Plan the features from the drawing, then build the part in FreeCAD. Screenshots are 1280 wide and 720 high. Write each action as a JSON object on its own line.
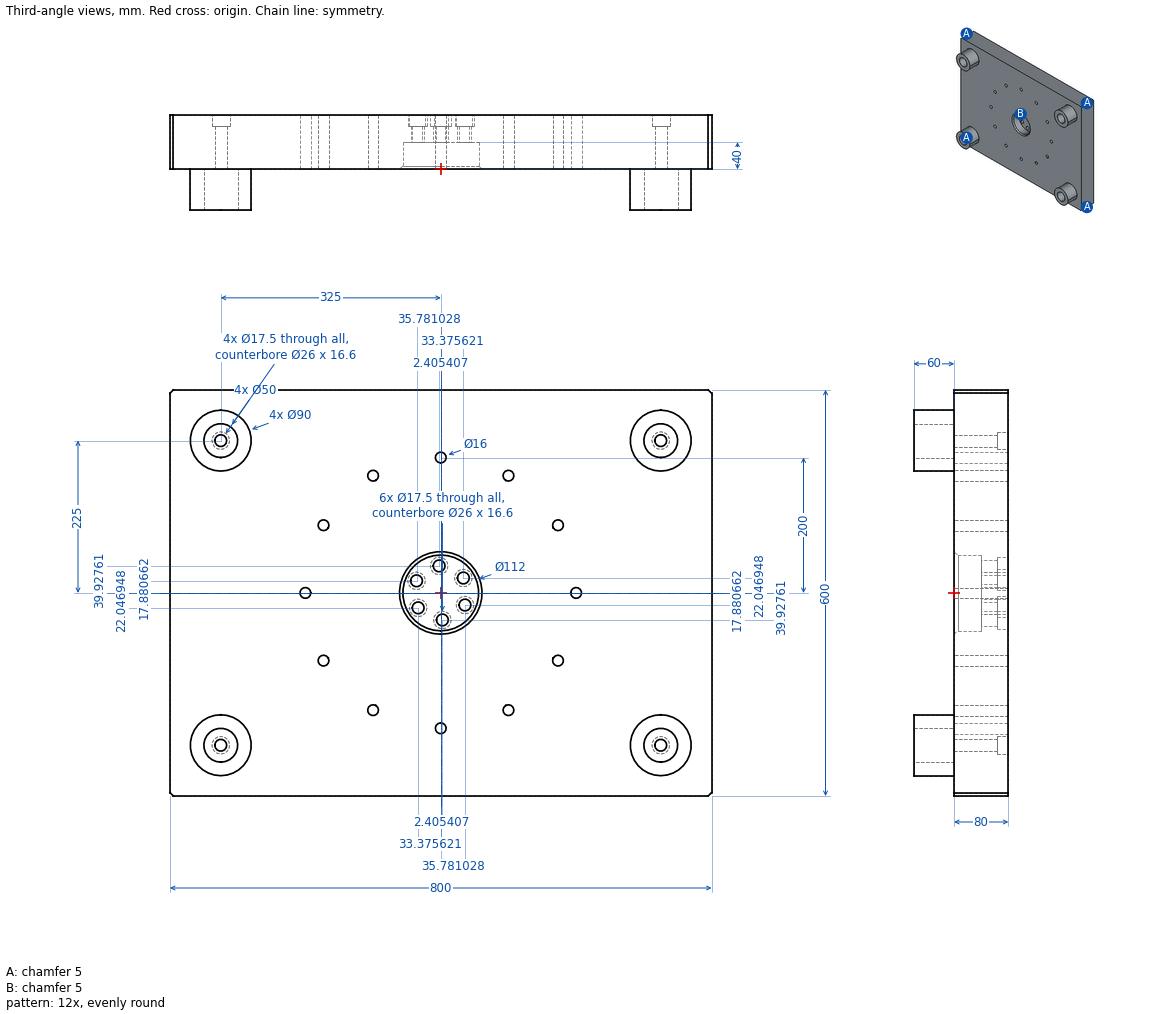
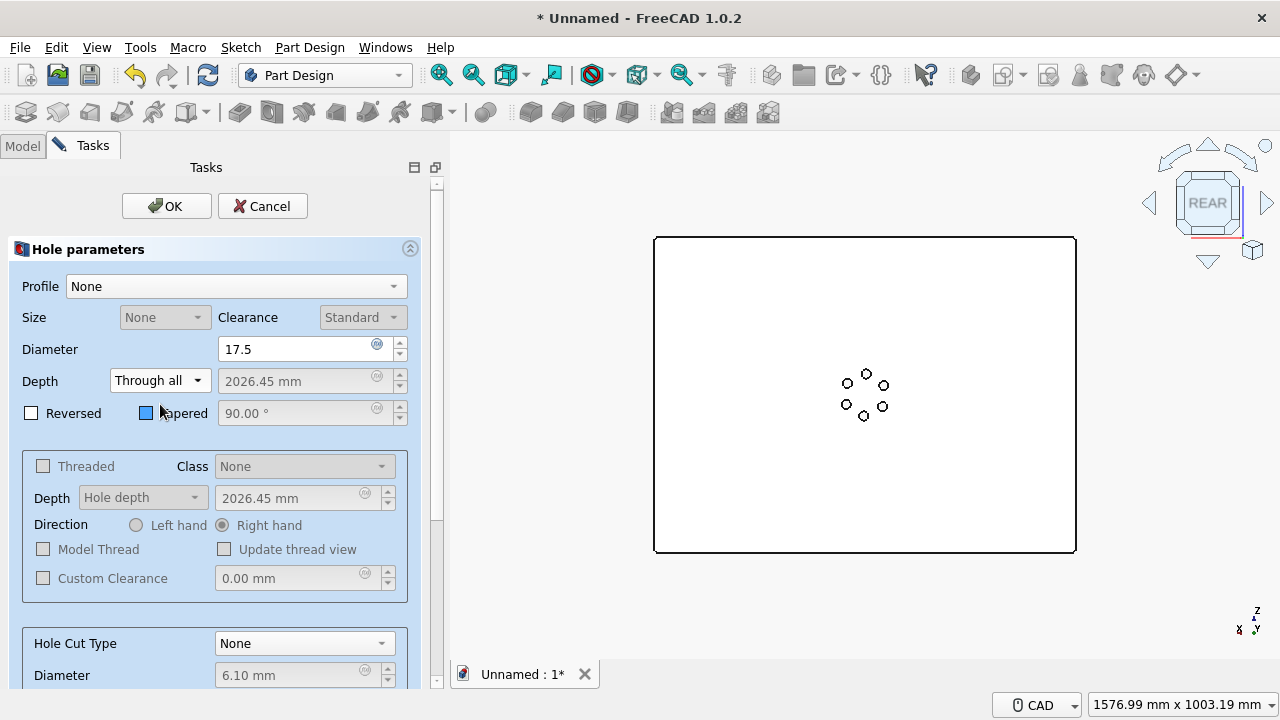
{"action": "left_click", "coordinate": [306, 644]}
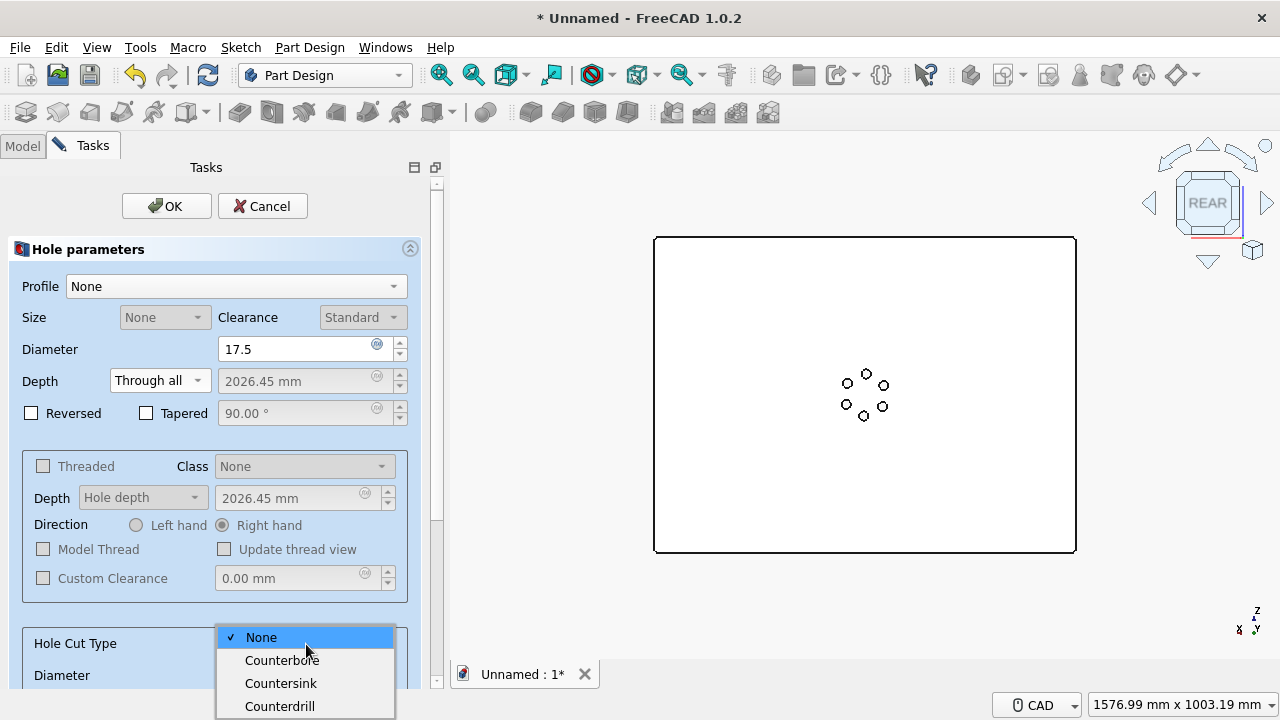
{"action": "left_click", "coordinate": [304, 660]}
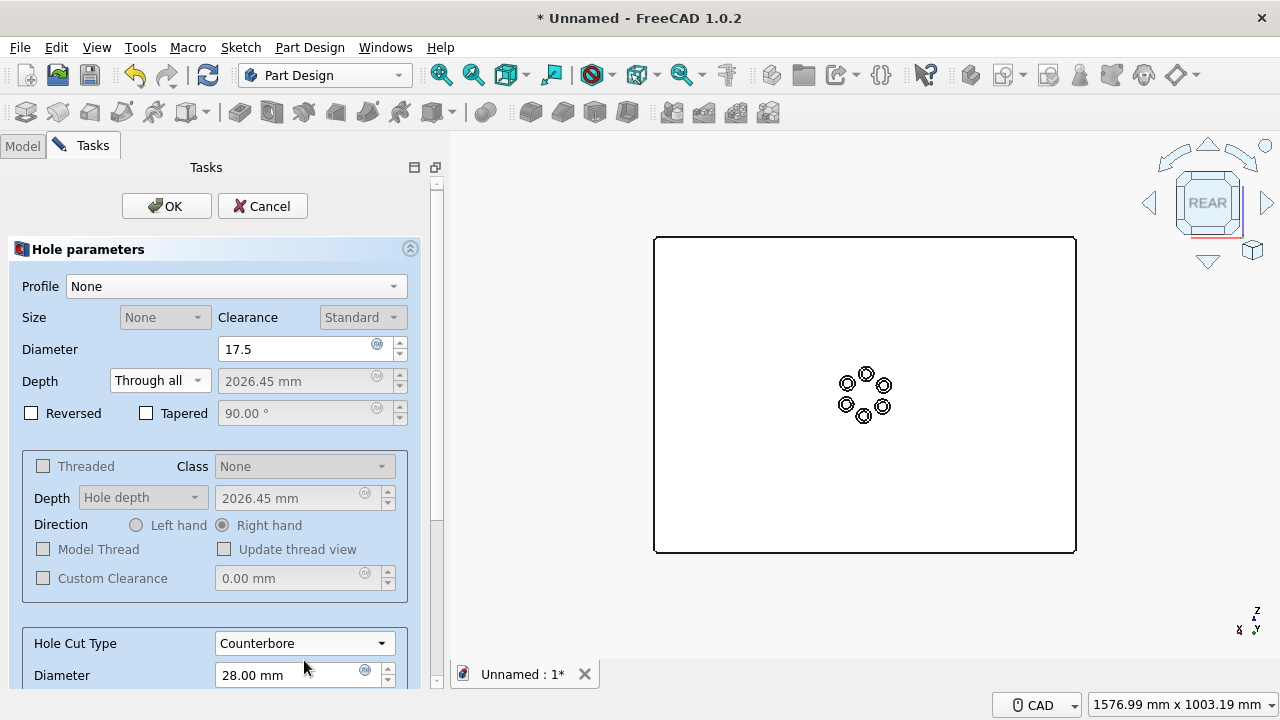
{"action": "triple_click", "coordinate": [298, 675]}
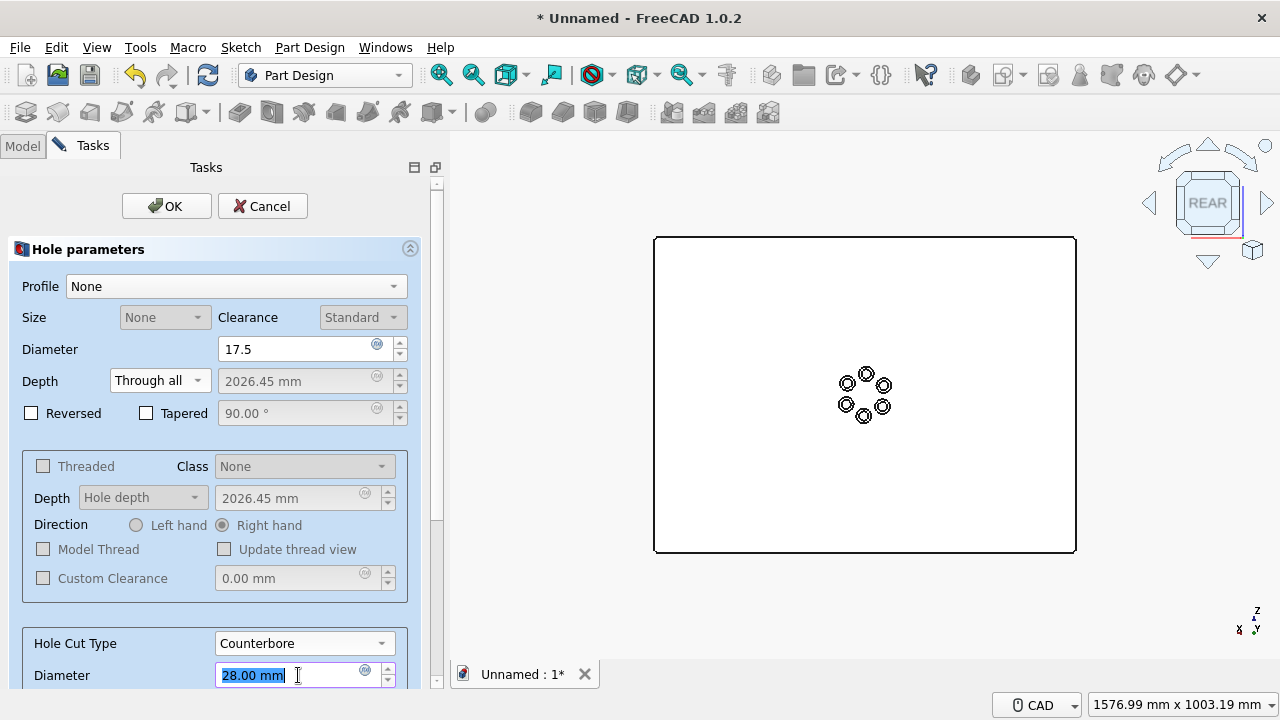
{"action": "type", "text": "26"}
{"action": "key", "text": "Tab"}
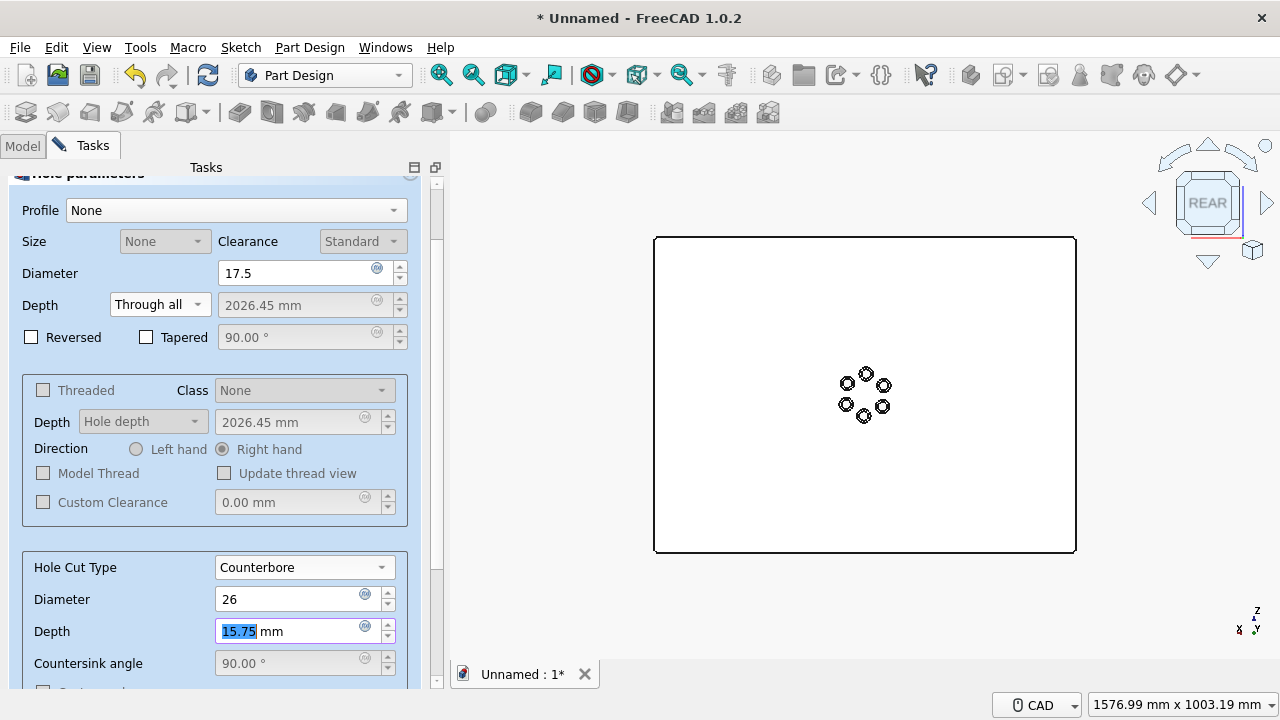
{"action": "type", "text": "16.6"}
{"action": "key", "text": "Tab"}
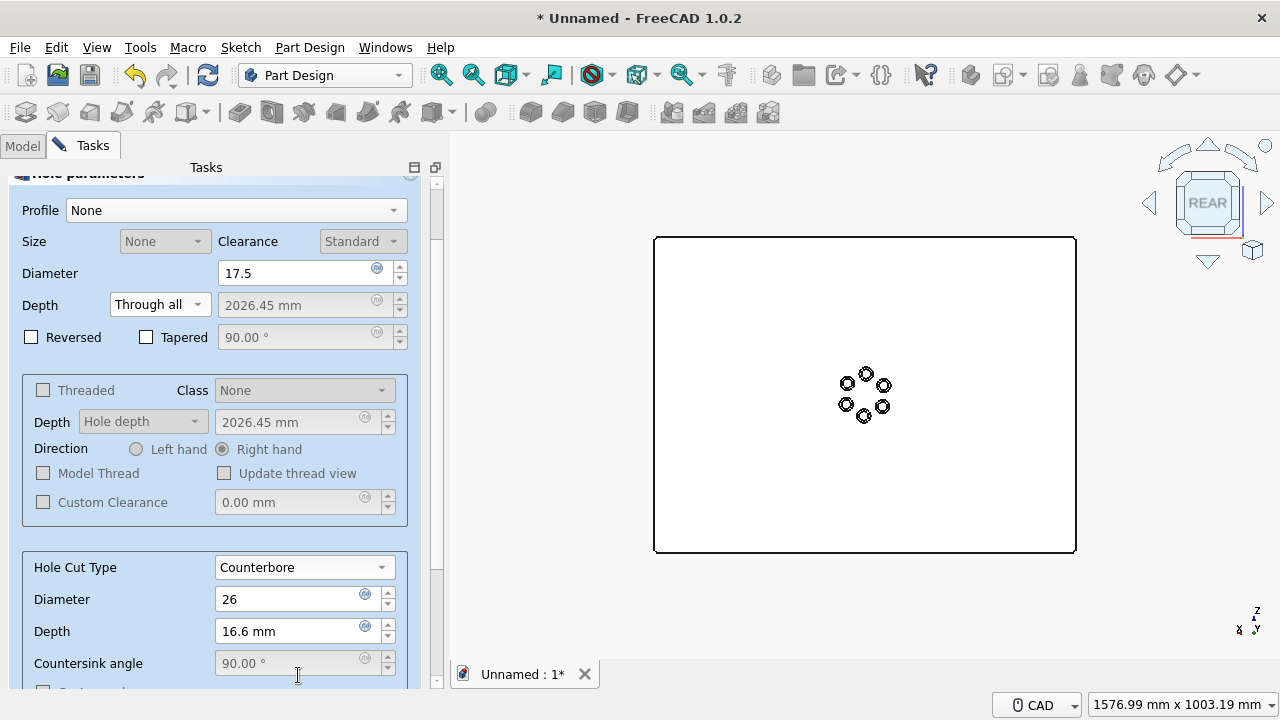
{"action": "scroll", "coordinate": [437, 432], "scroll_direction": "up", "scroll_amount": 3}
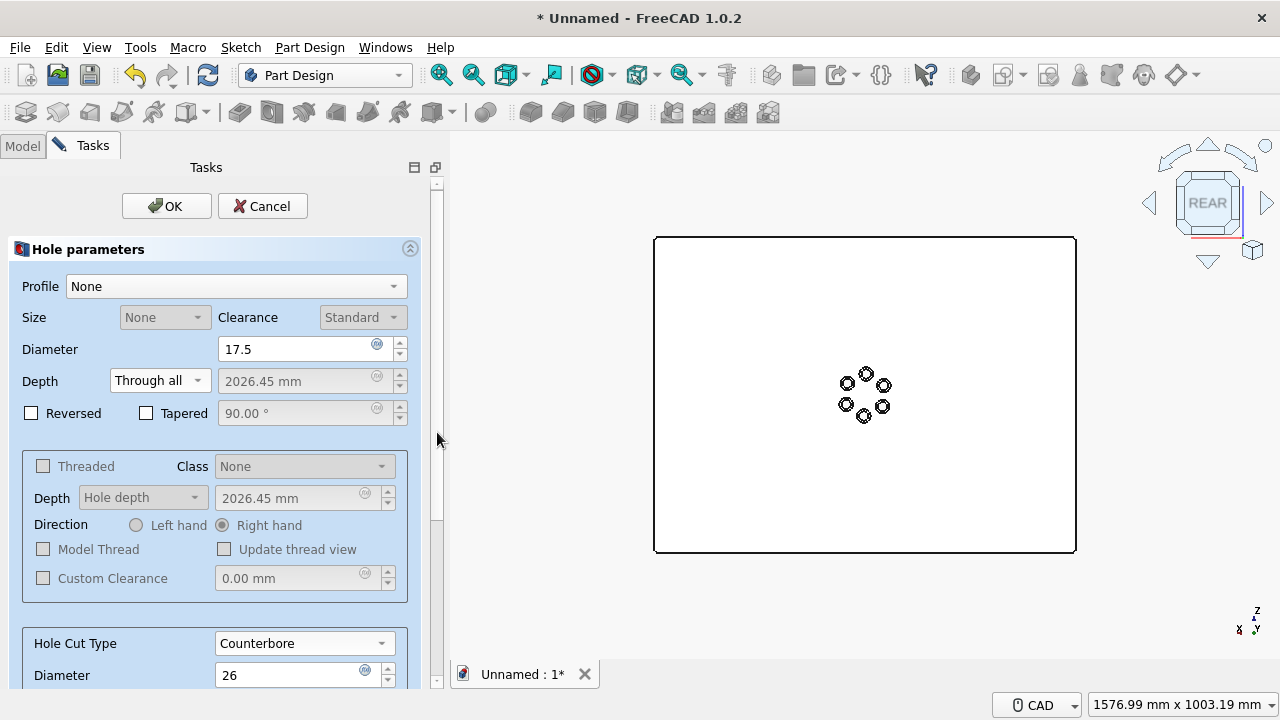
{"action": "left_click", "coordinate": [167, 206]}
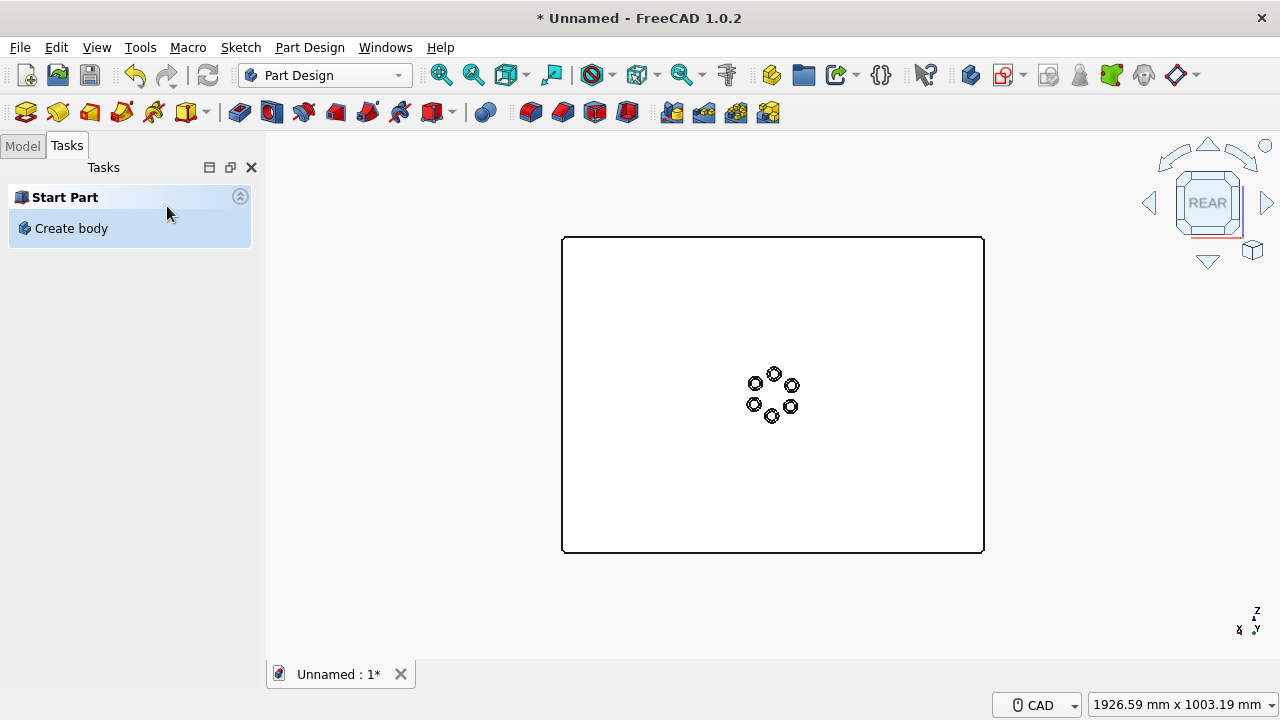
{"action": "key", "text": "0"}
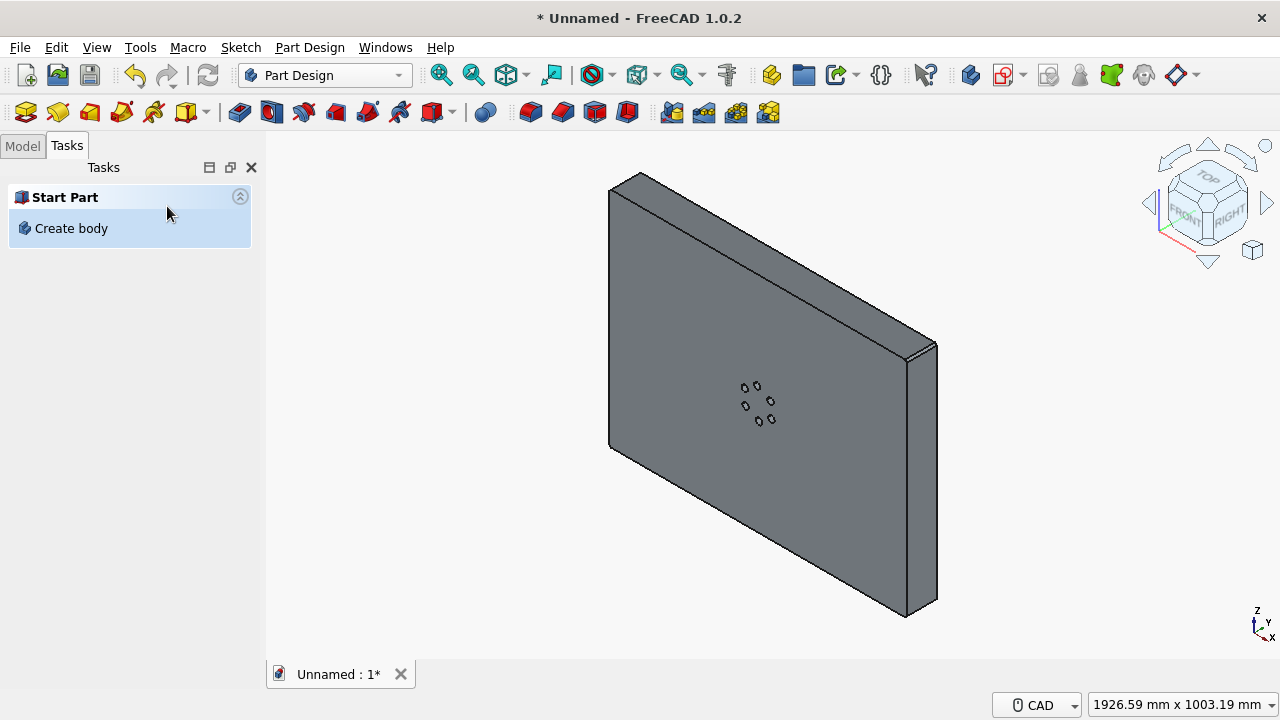
{"action": "left_click", "coordinate": [843, 415]}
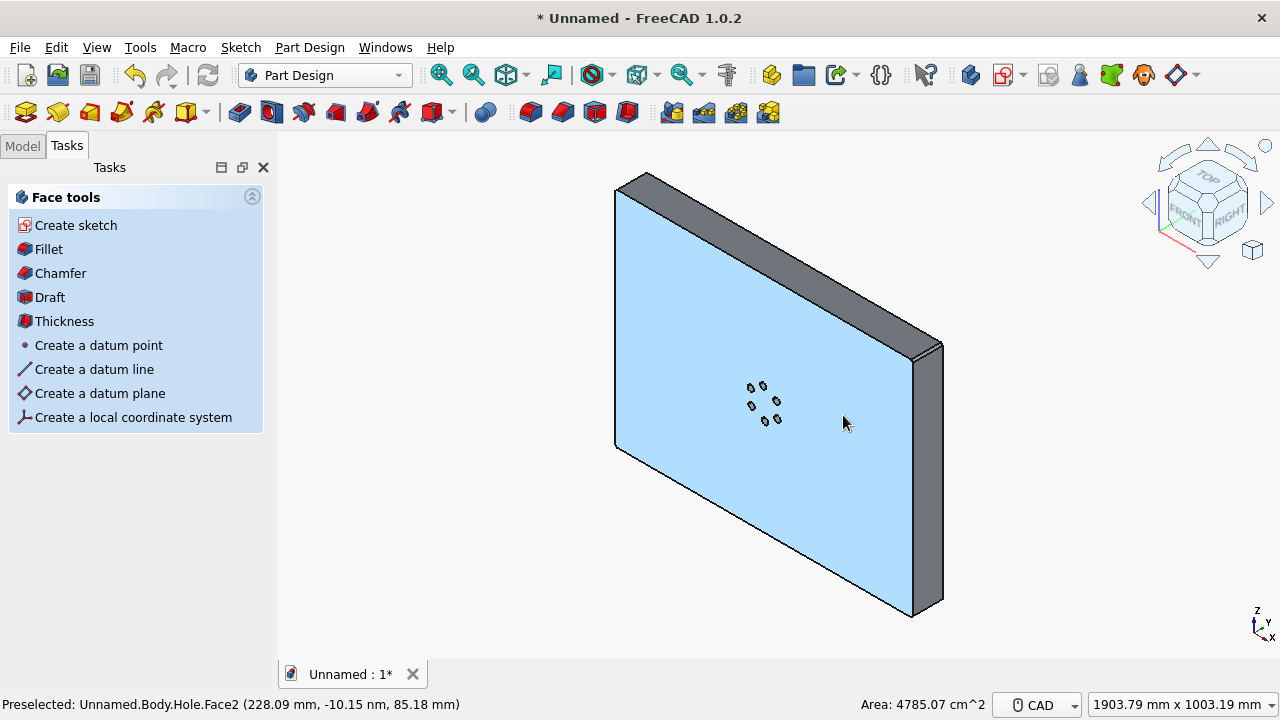
{"action": "left_click", "coordinate": [1004, 76]}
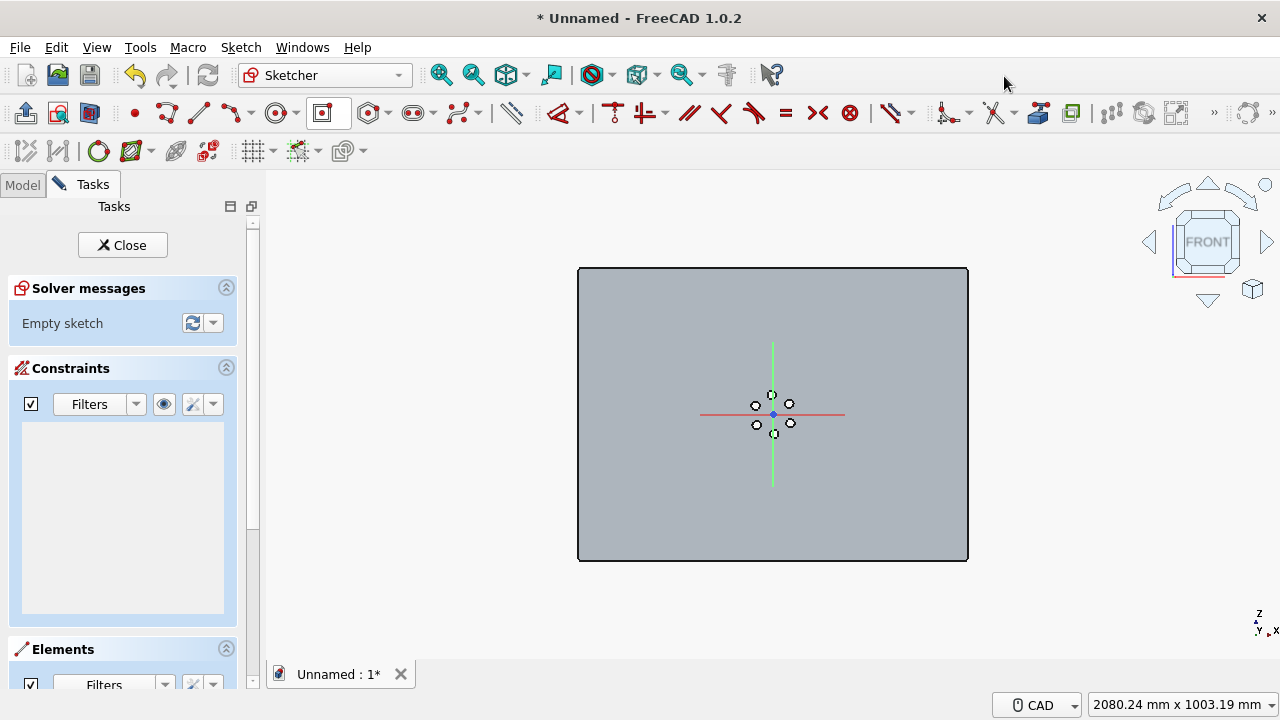
{"action": "scroll", "coordinate": [787, 415], "scroll_direction": "up", "scroll_amount": 9}